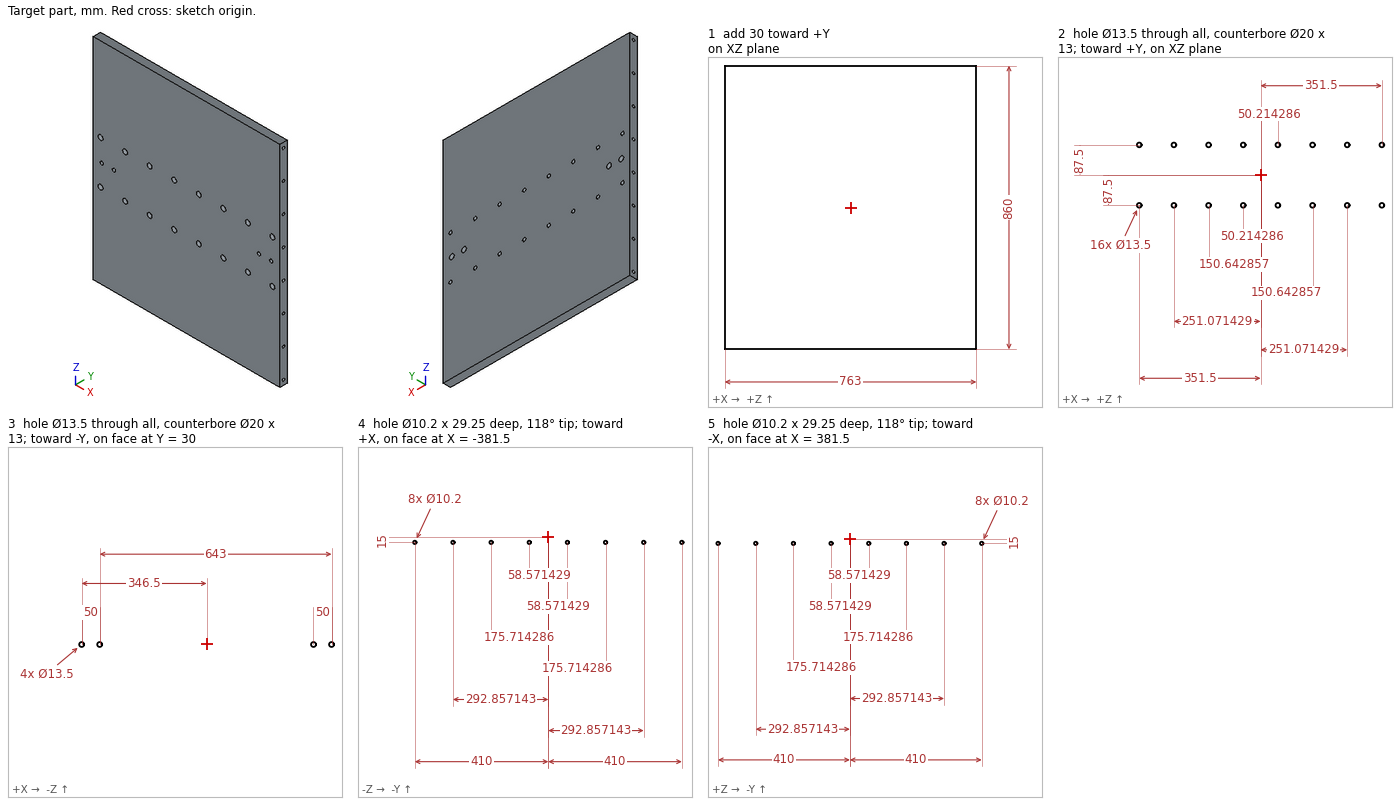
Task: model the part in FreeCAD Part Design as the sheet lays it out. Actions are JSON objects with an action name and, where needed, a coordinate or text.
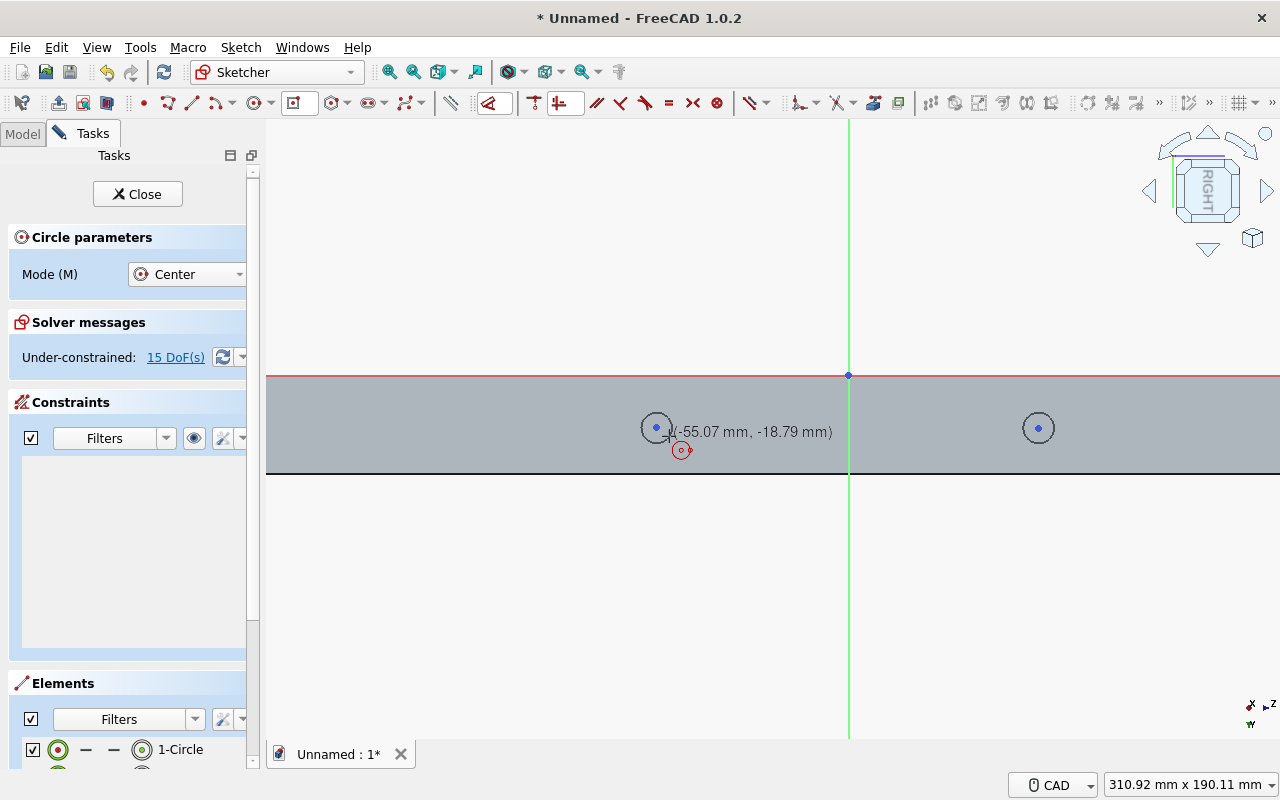
{"action": "scroll", "coordinate": [668, 434], "scroll_direction": "down", "scroll_amount": 8}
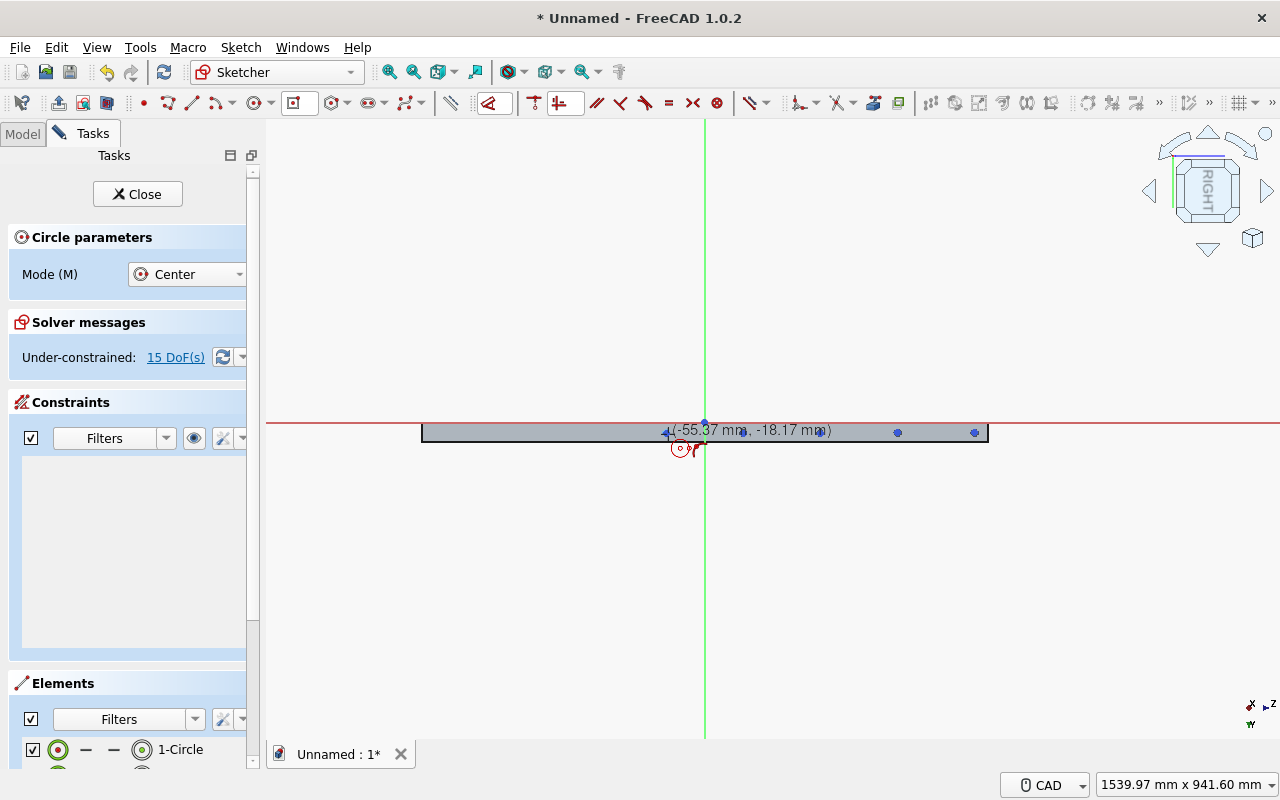
{"action": "scroll", "coordinate": [589, 433], "scroll_direction": "up", "scroll_amount": 10}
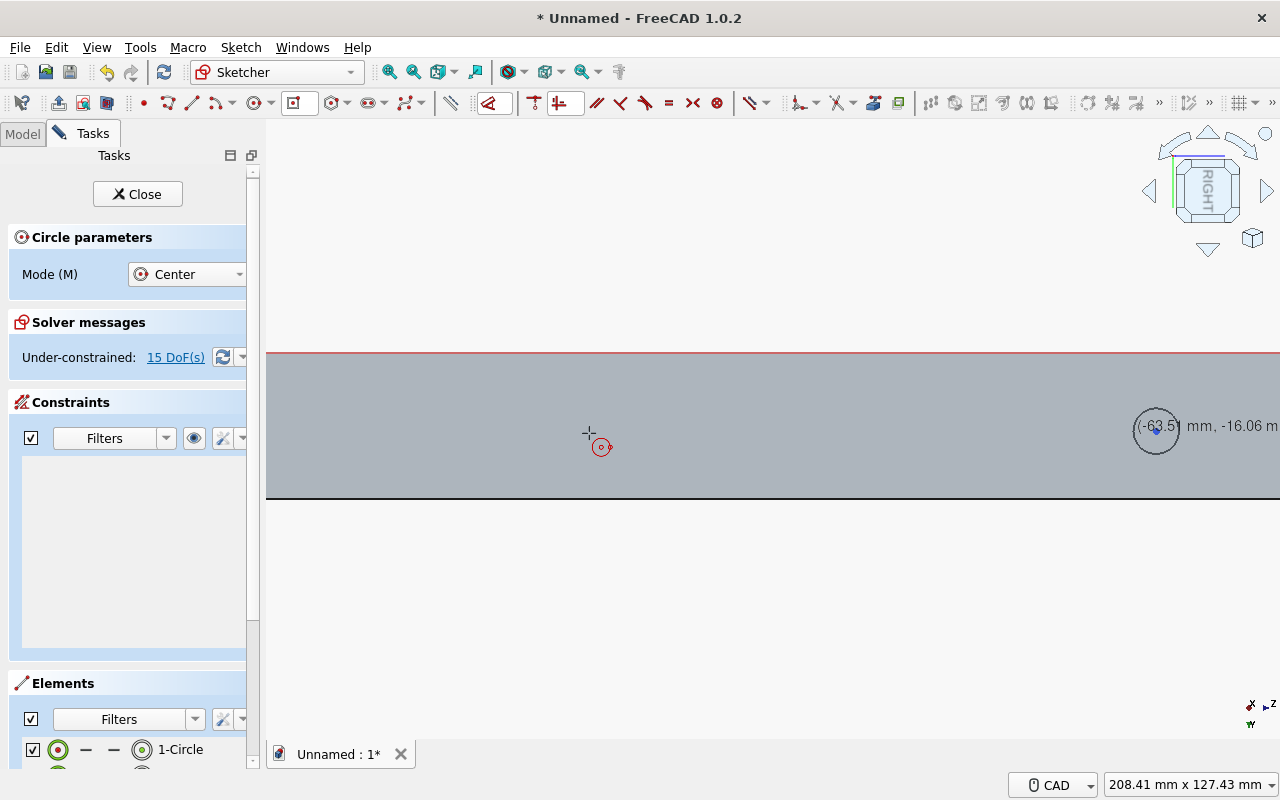
{"action": "scroll", "coordinate": [589, 433], "scroll_direction": "down", "scroll_amount": 10}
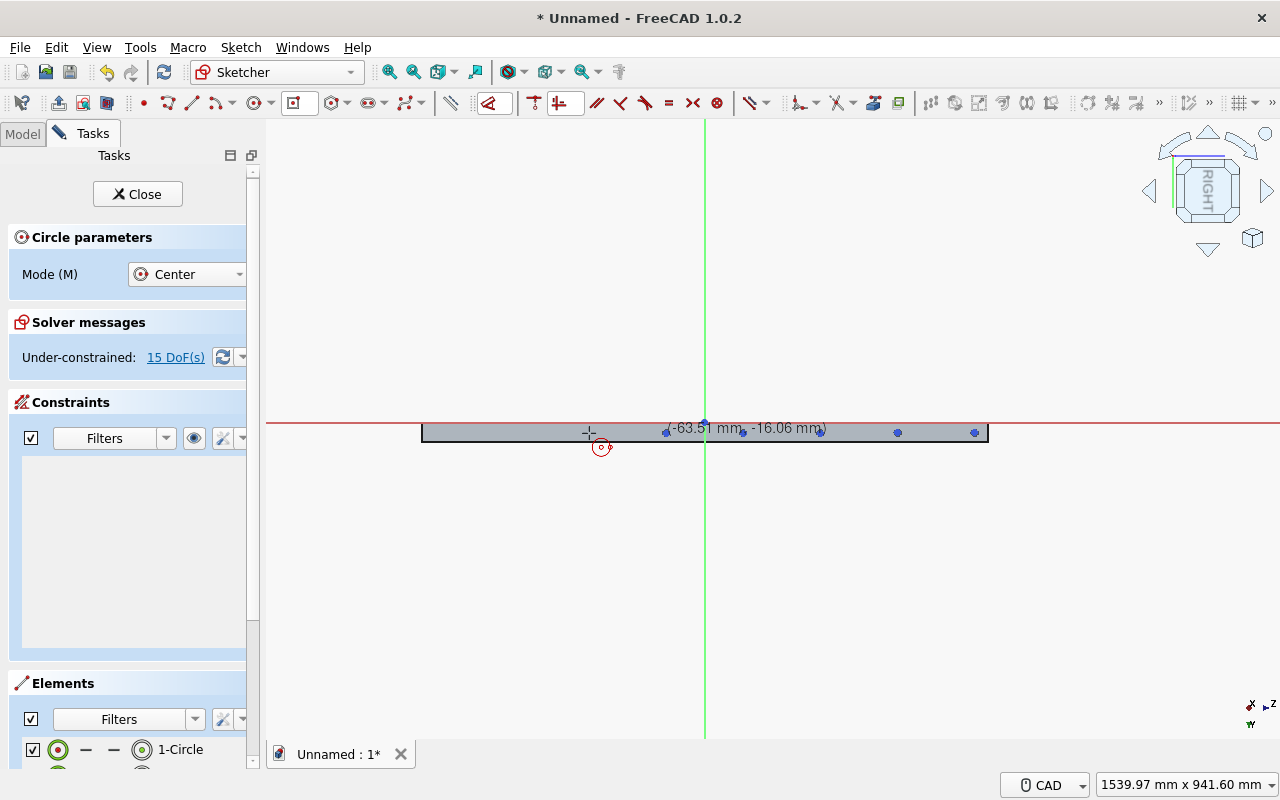
{"action": "scroll", "coordinate": [589, 433], "scroll_direction": "up", "scroll_amount": 3}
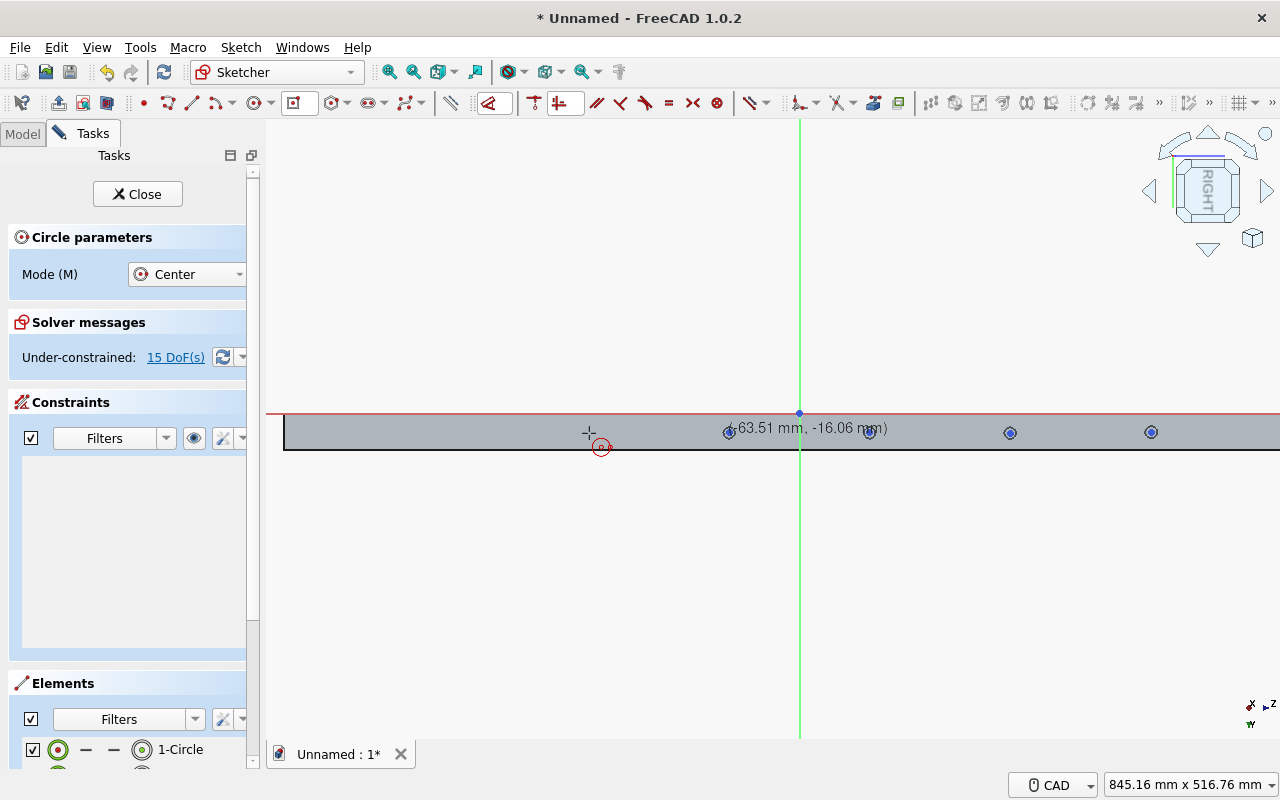
{"action": "left_click", "coordinate": [589, 432]}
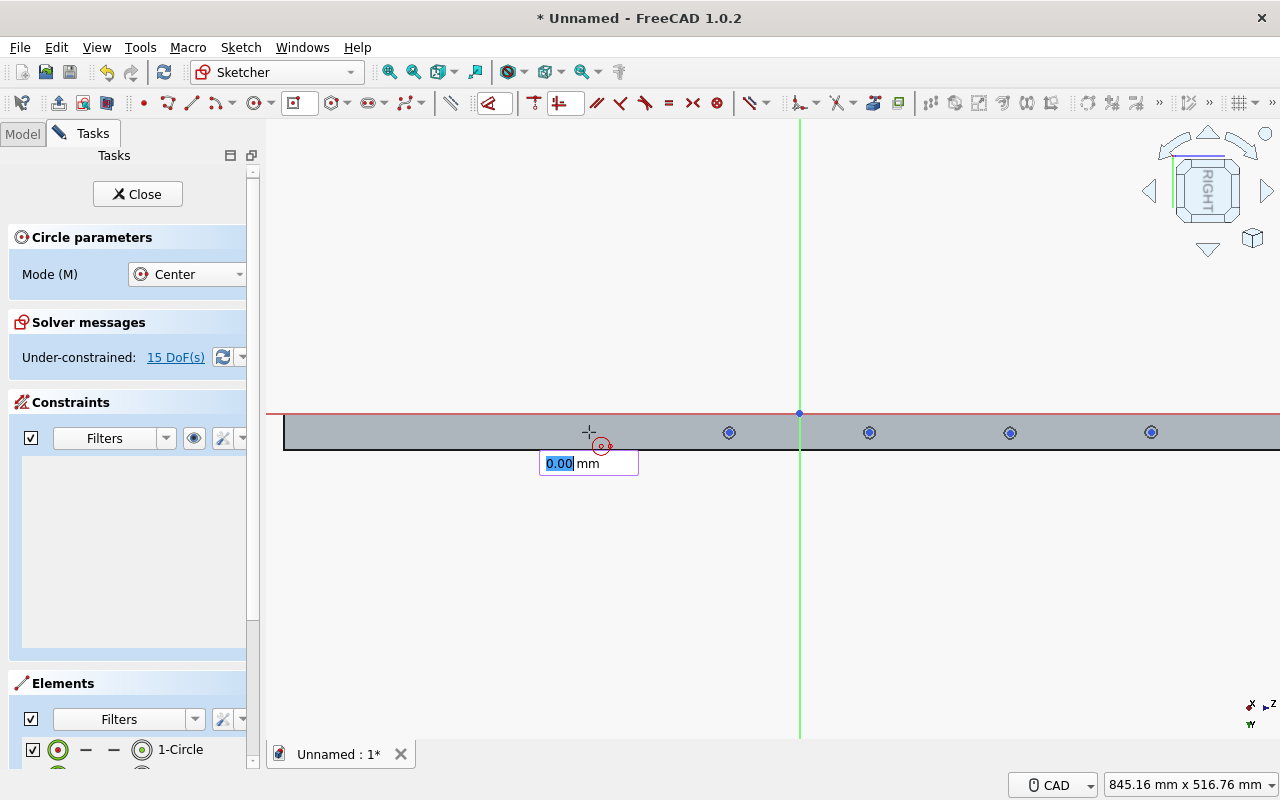
{"action": "scroll", "coordinate": [593, 436], "scroll_direction": "up", "scroll_amount": 5}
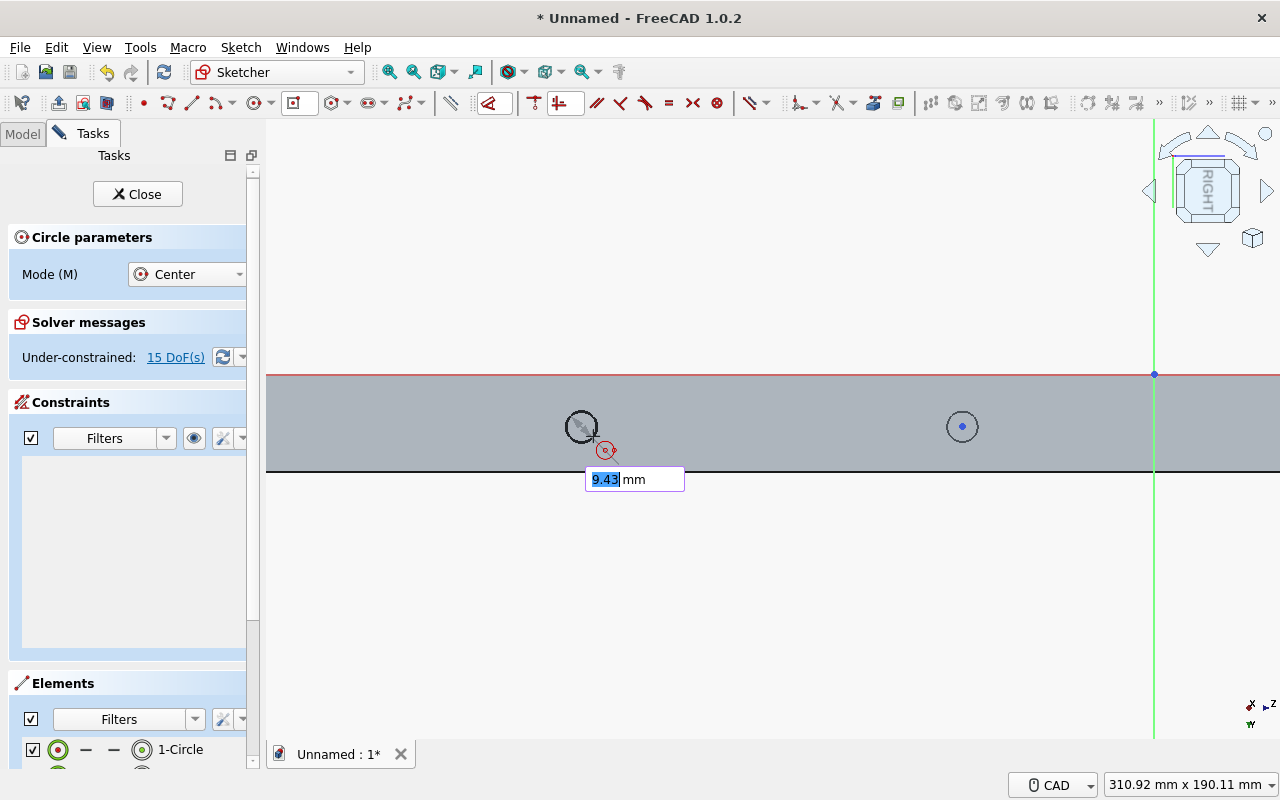
{"action": "left_click", "coordinate": [593, 435]}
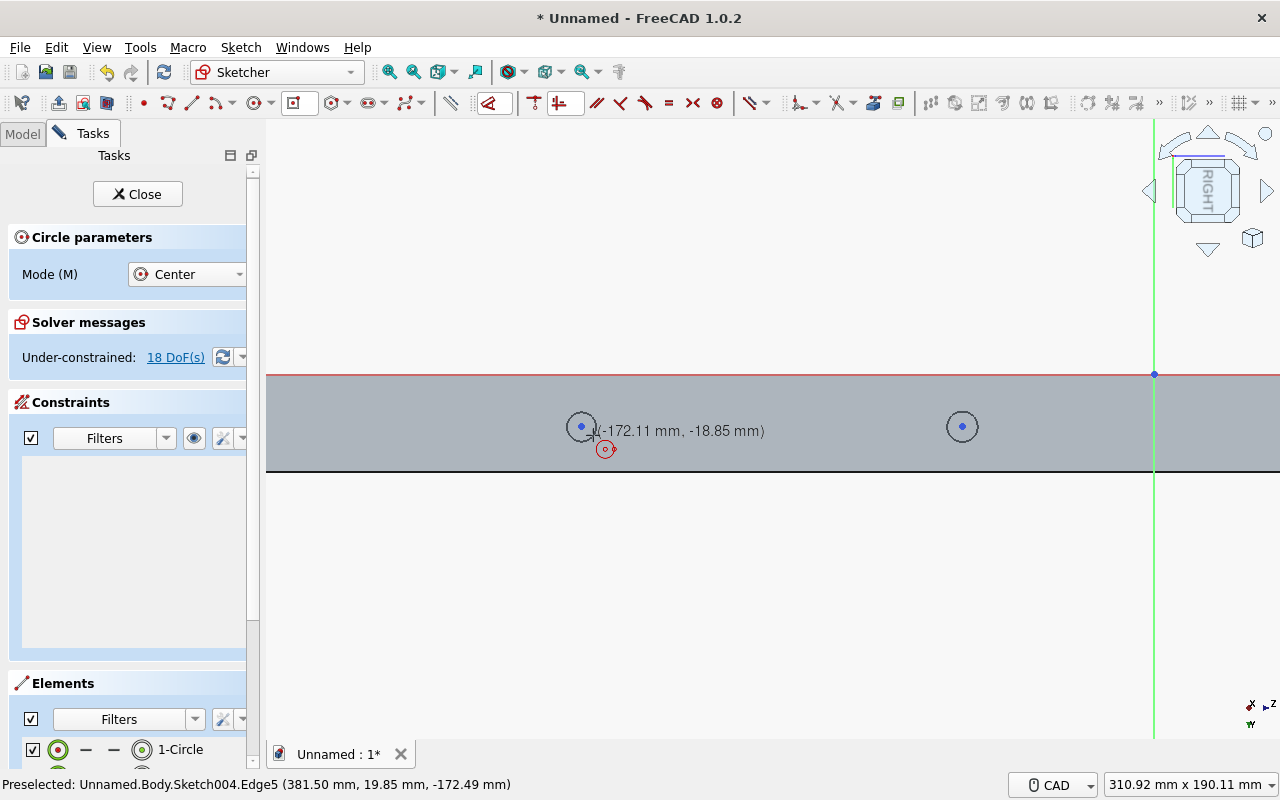
{"action": "scroll", "coordinate": [591, 434], "scroll_direction": "down", "scroll_amount": 8}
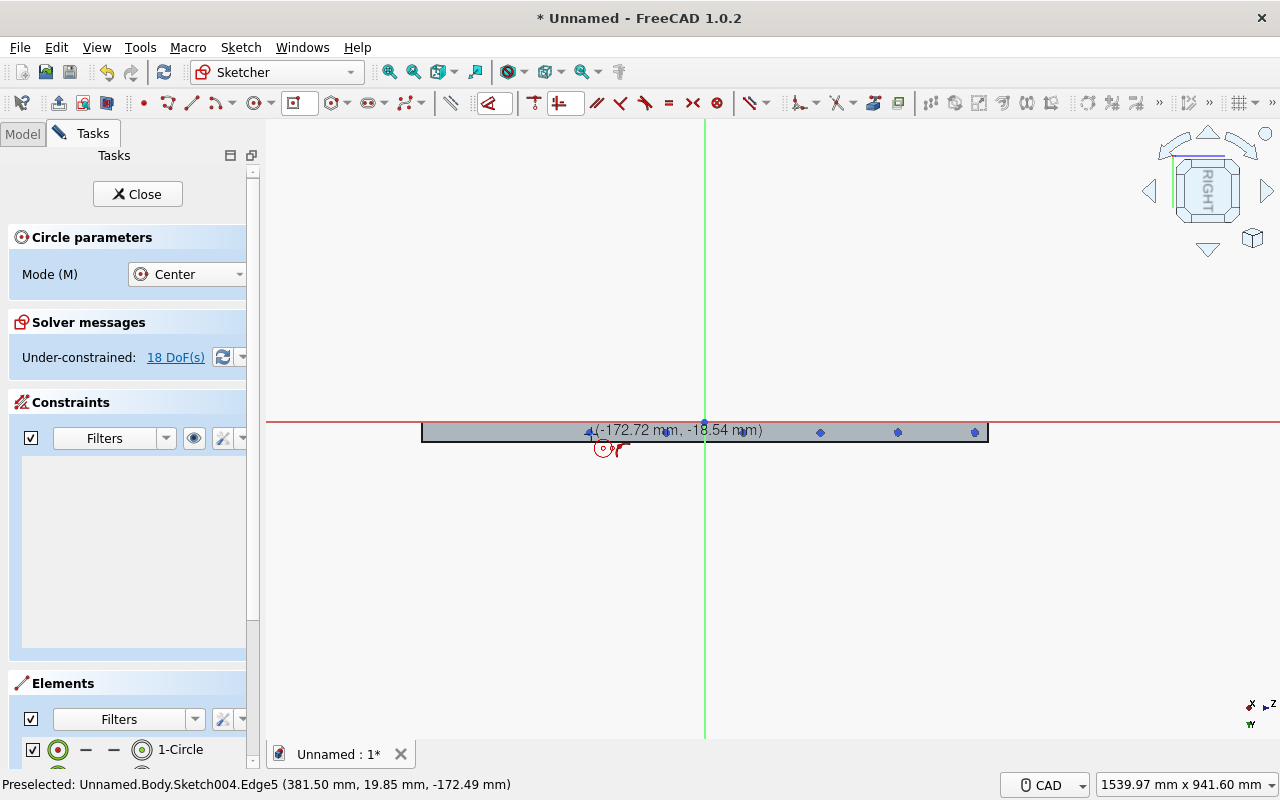
{"action": "scroll", "coordinate": [512, 432], "scroll_direction": "up", "scroll_amount": 10}